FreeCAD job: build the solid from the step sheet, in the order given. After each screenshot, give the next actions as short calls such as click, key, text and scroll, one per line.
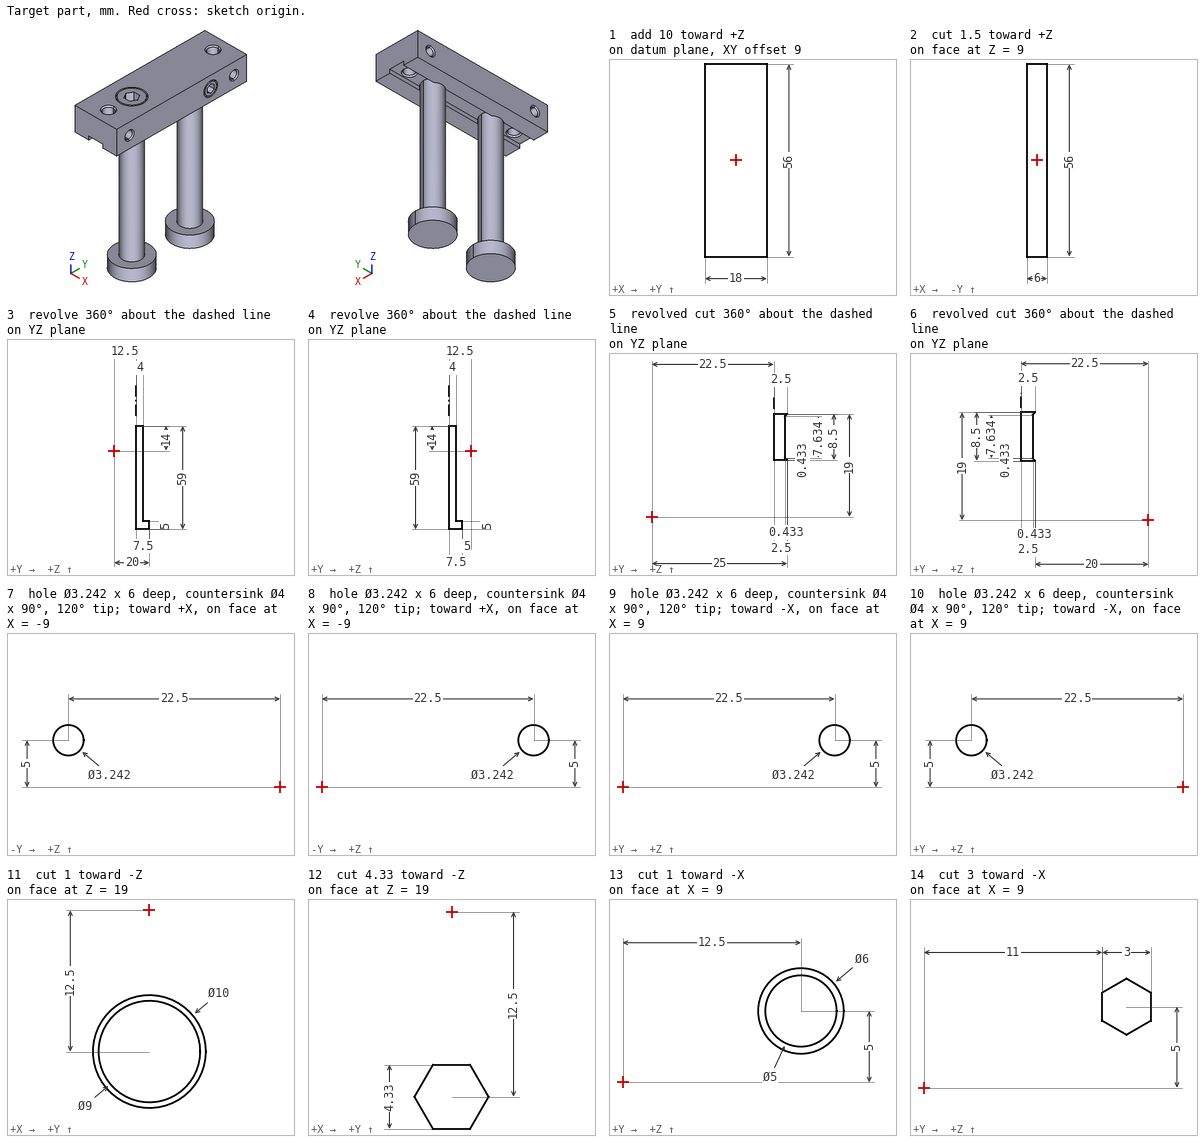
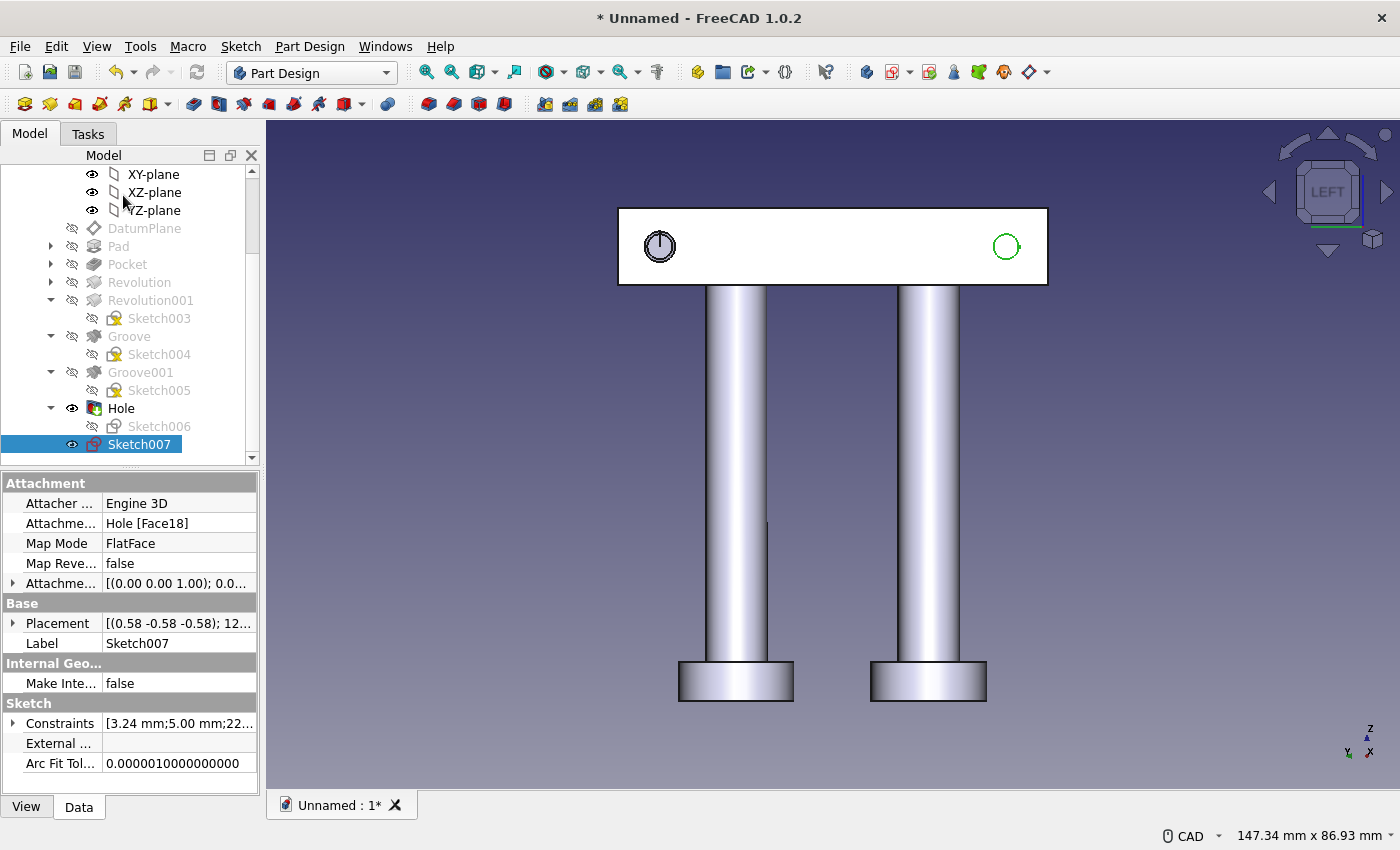
click(219, 104)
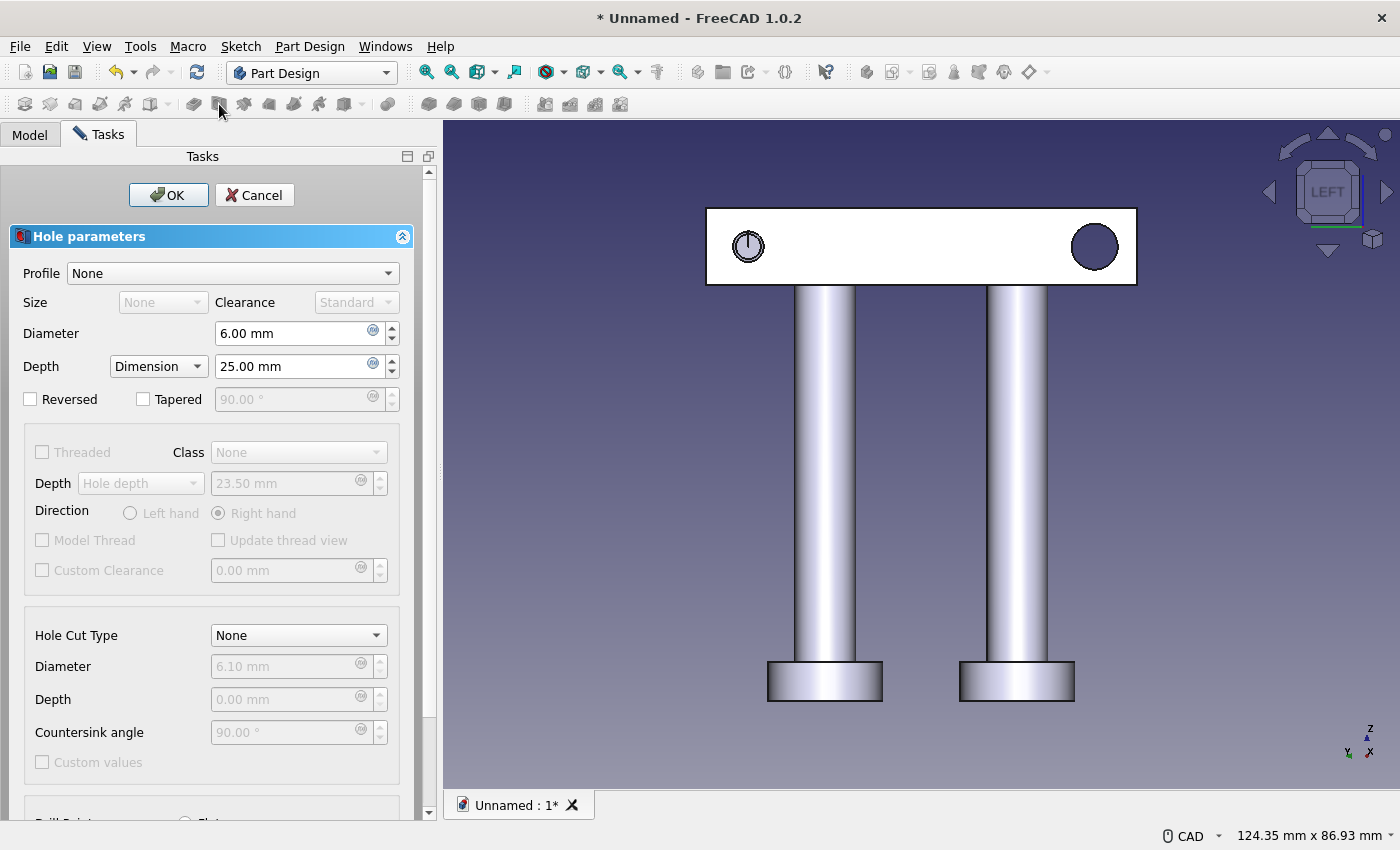
triple_click(300, 334)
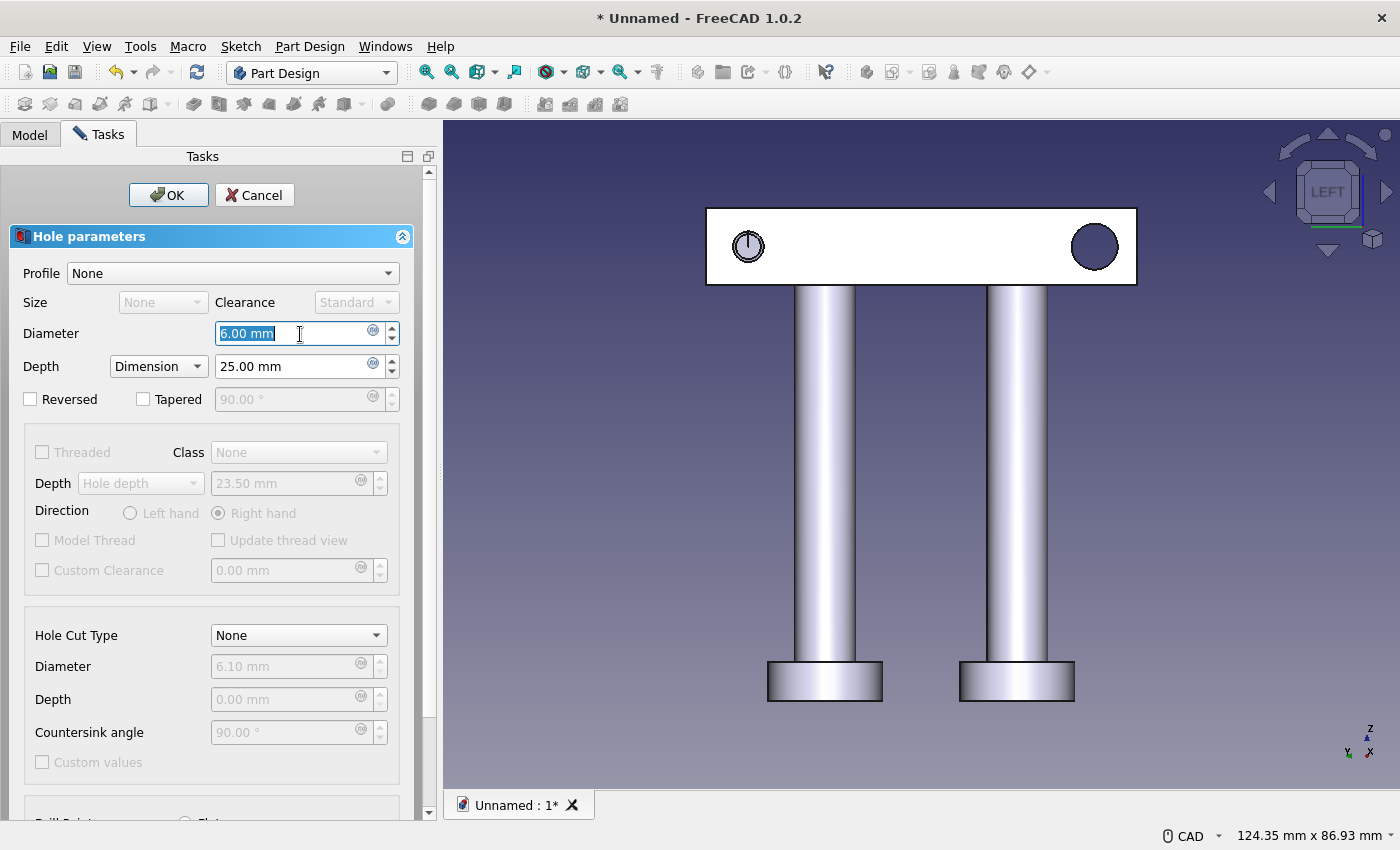
text(3.242)
key(Tab)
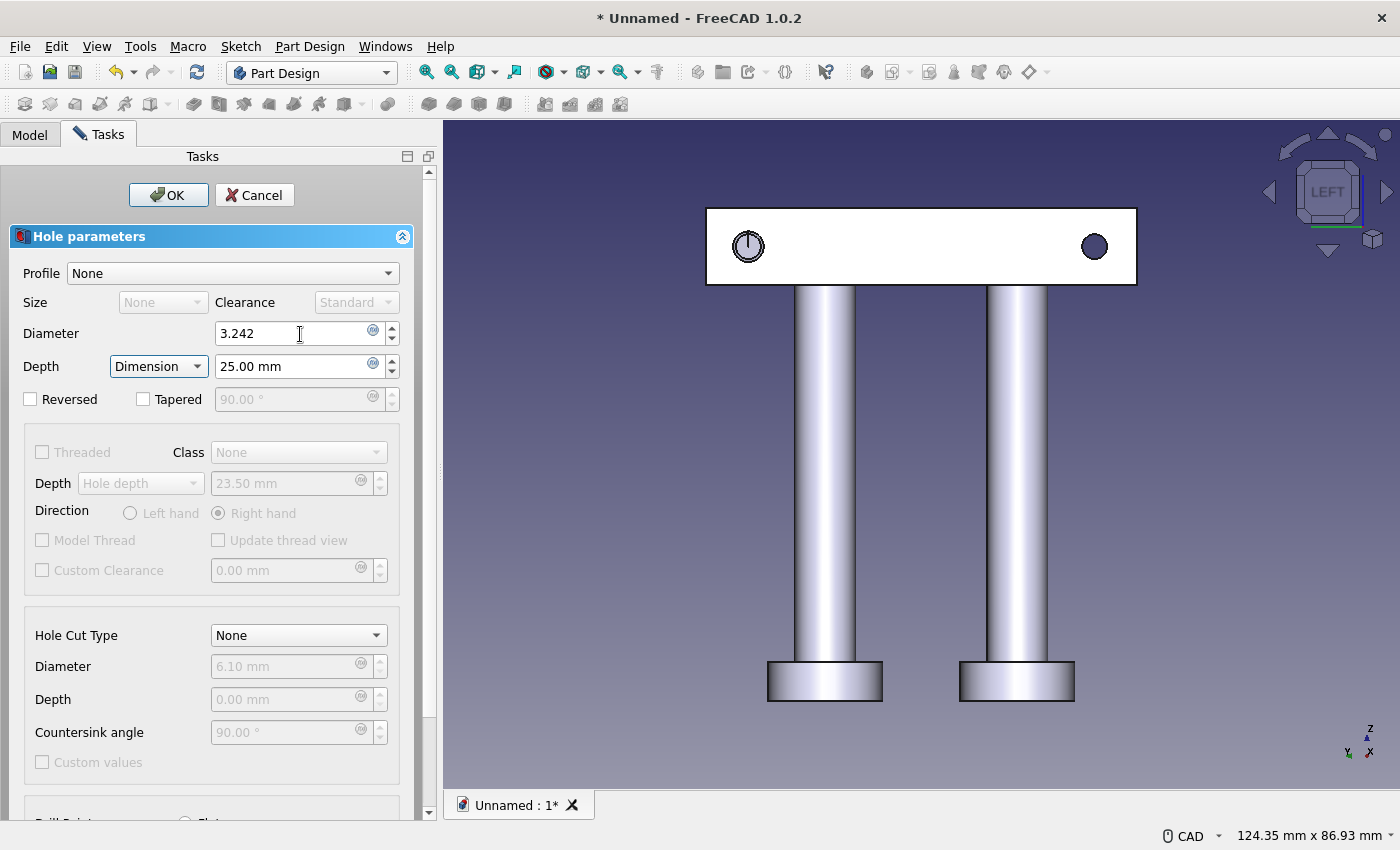
triple_click(300, 366)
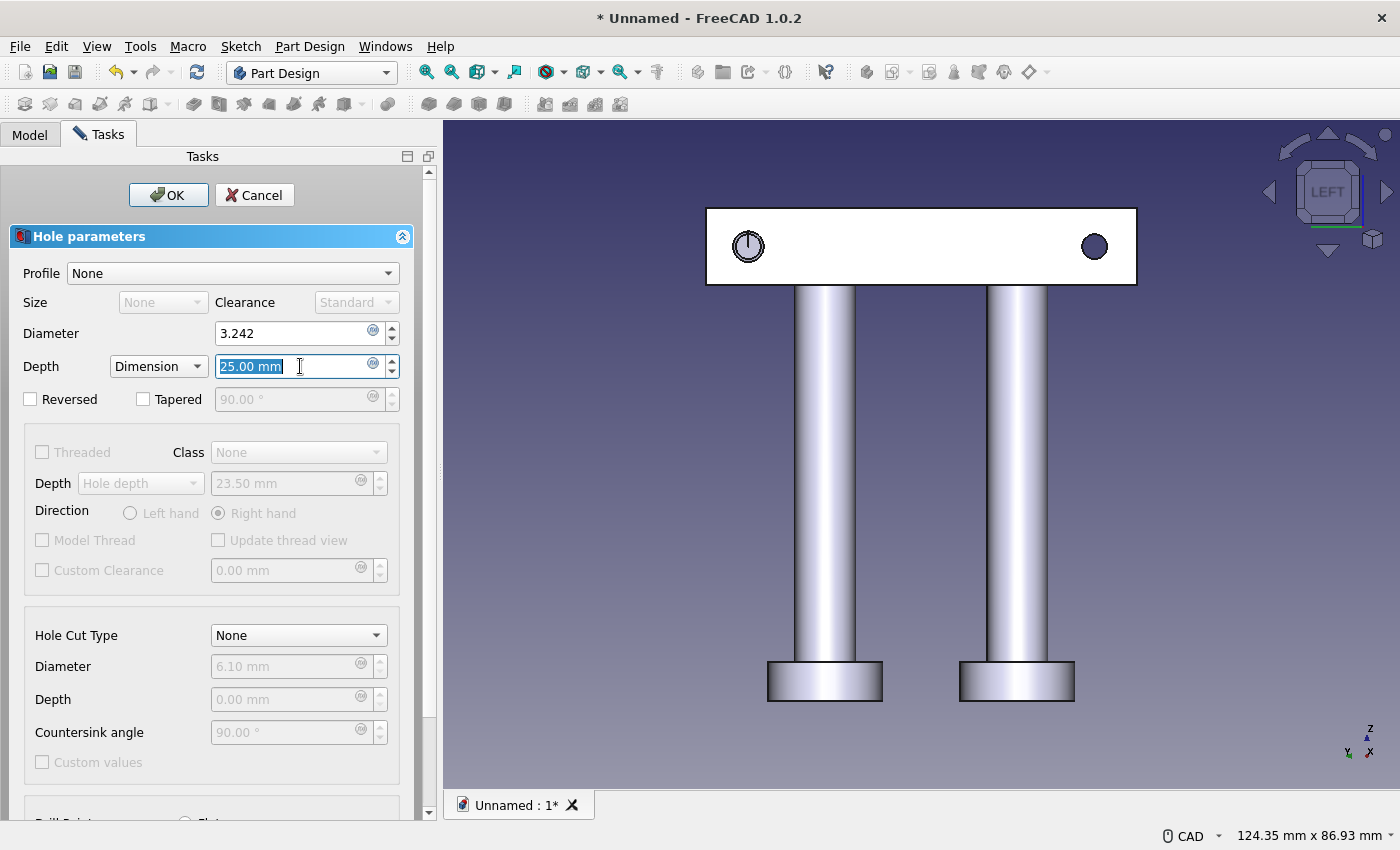
text(6)
key(Tab)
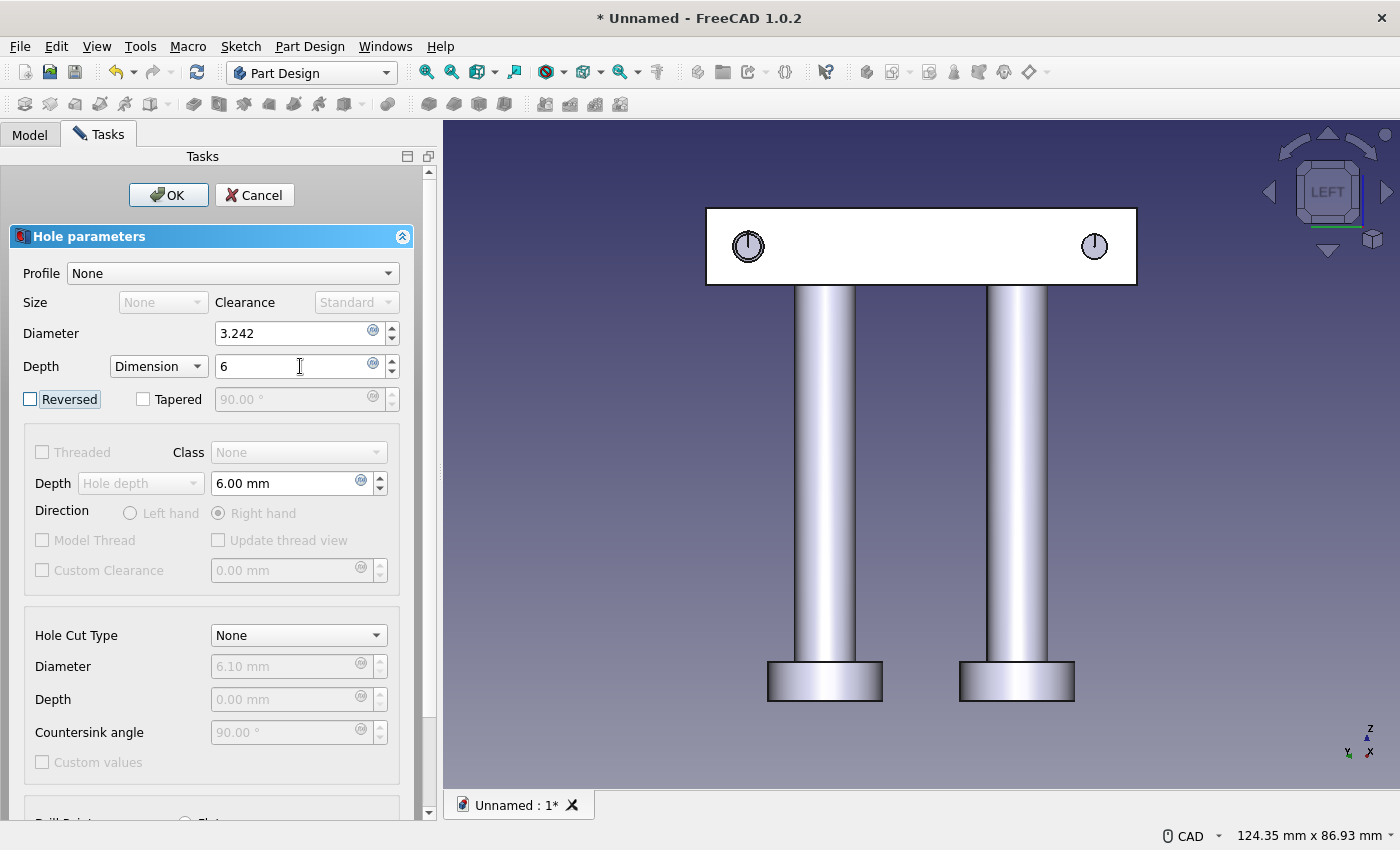
click(300, 636)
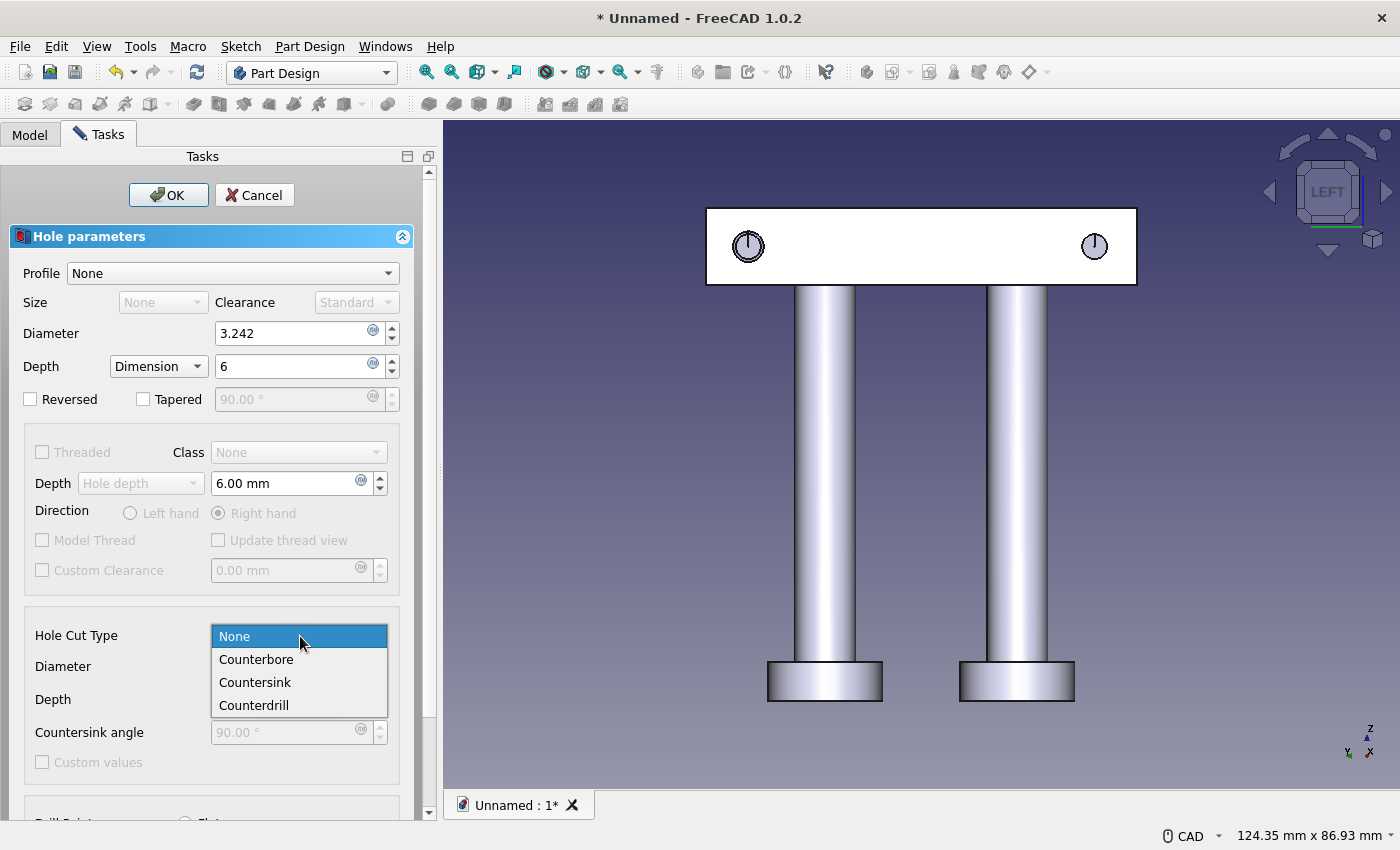
click(298, 682)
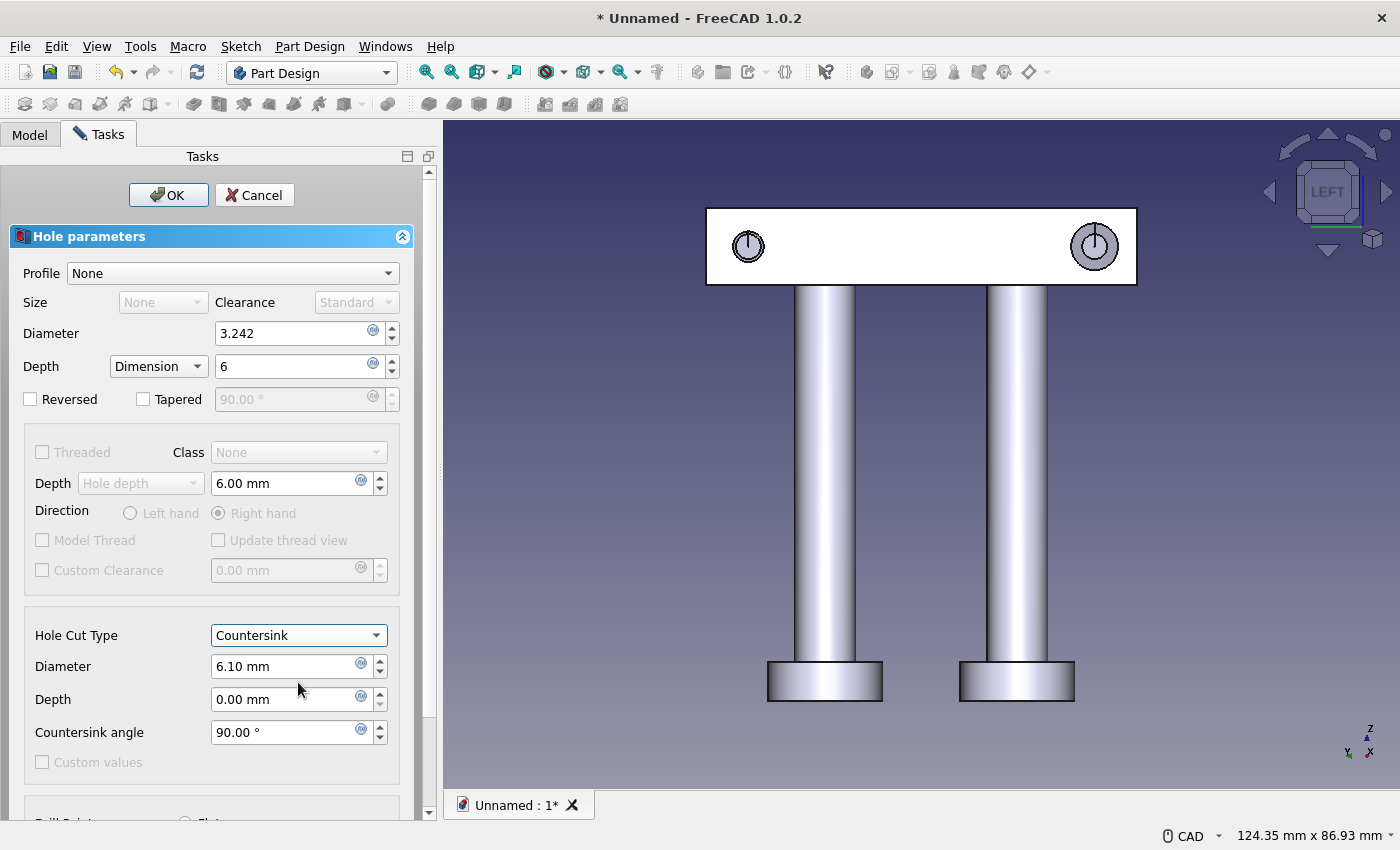
triple_click(292, 666)